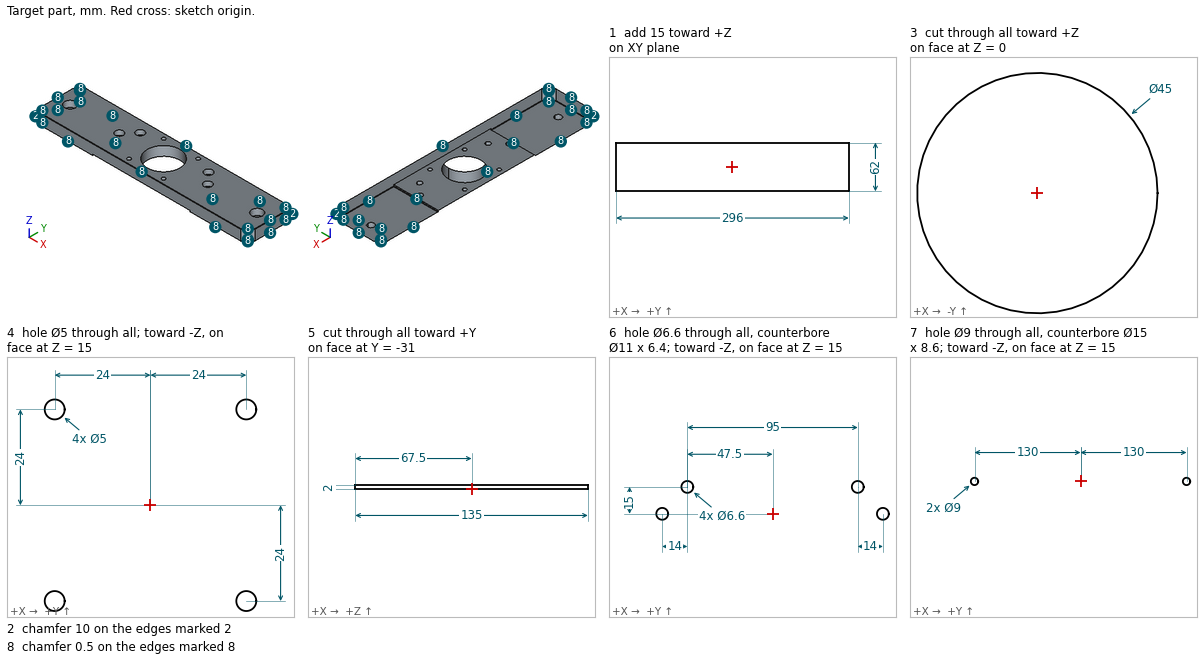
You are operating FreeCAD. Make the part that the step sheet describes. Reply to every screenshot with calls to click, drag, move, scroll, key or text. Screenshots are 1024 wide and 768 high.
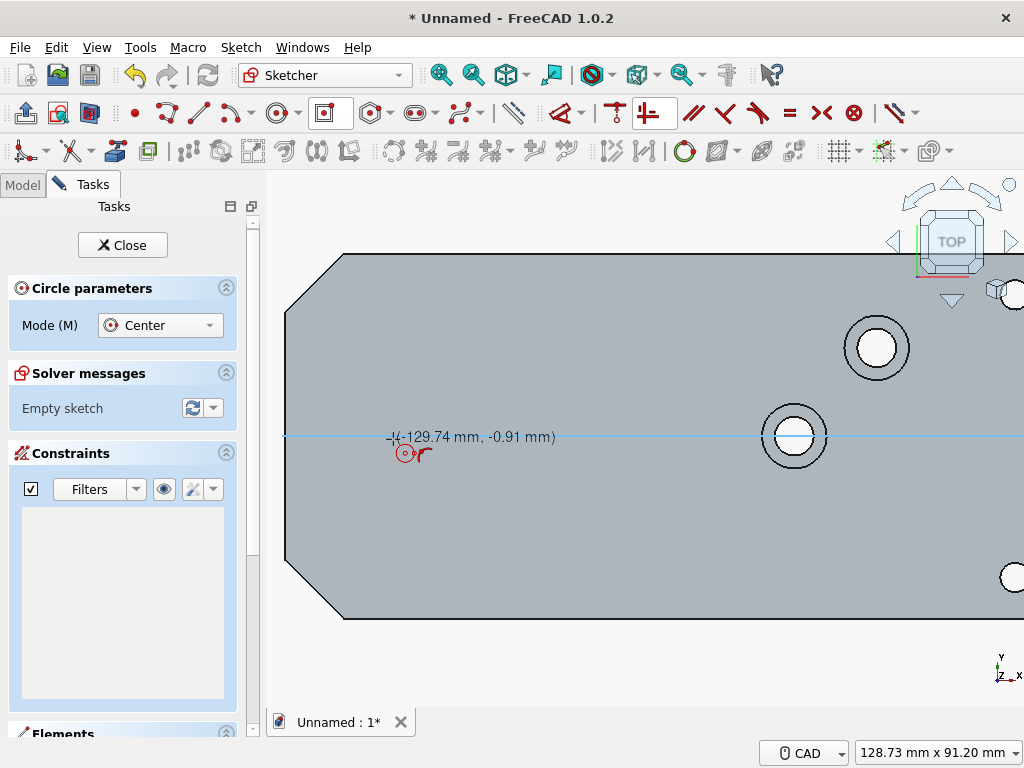
scroll(387, 439, down, 7)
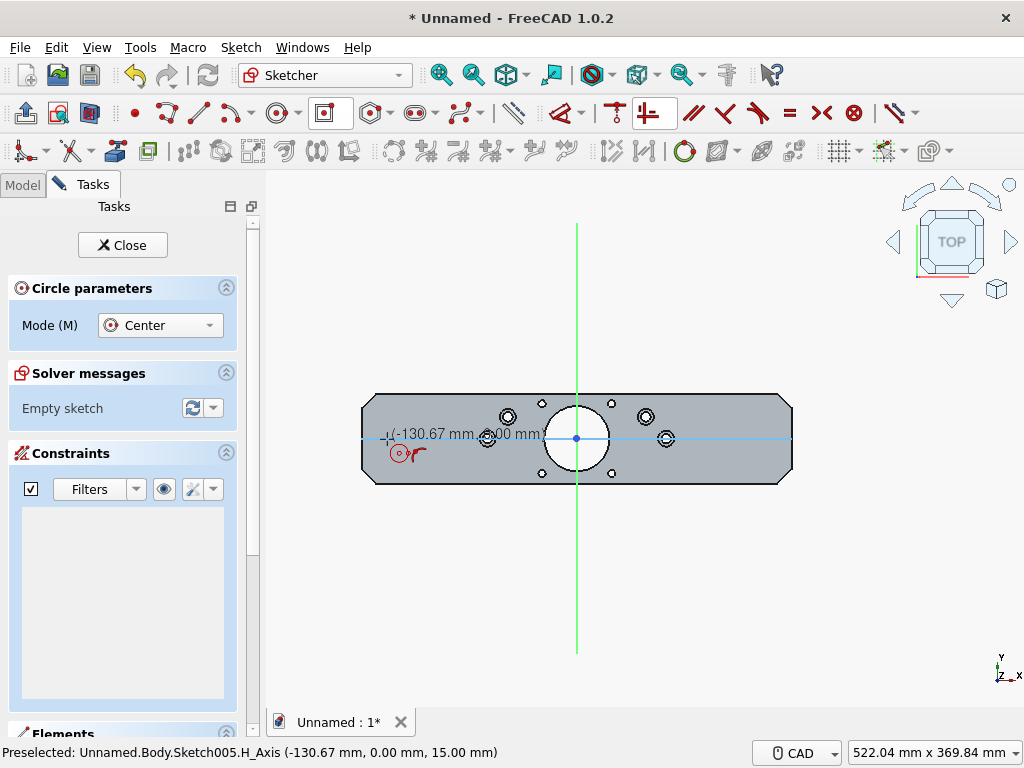
click(388, 439)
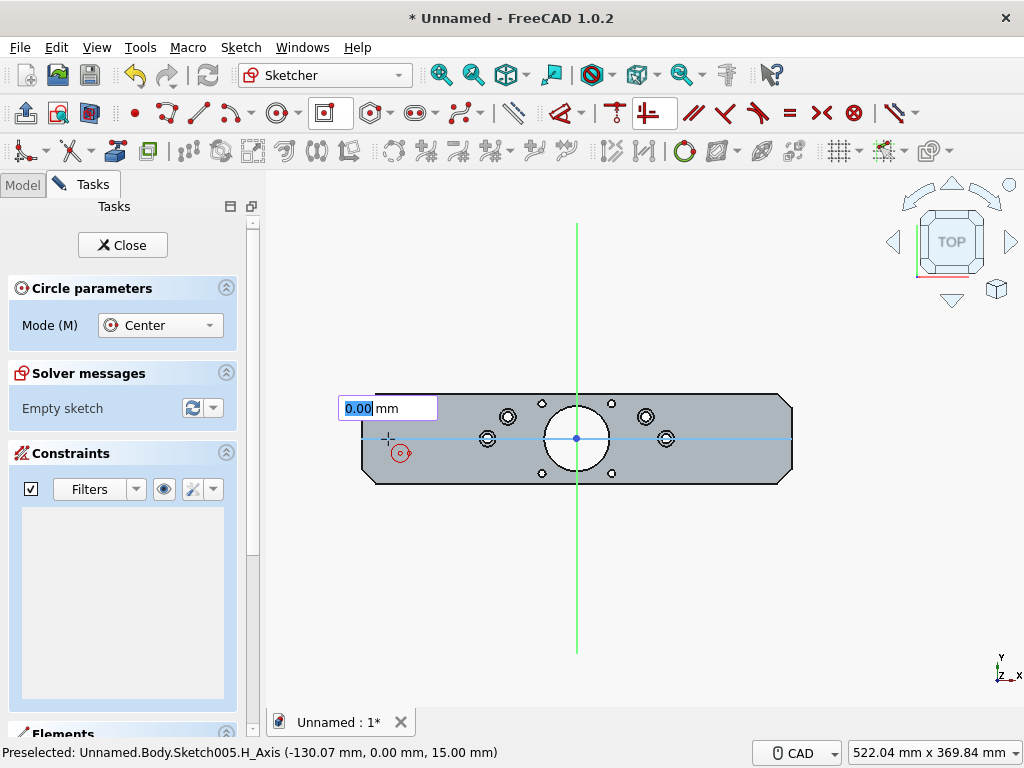
scroll(386, 445, up, 5)
move(385, 444)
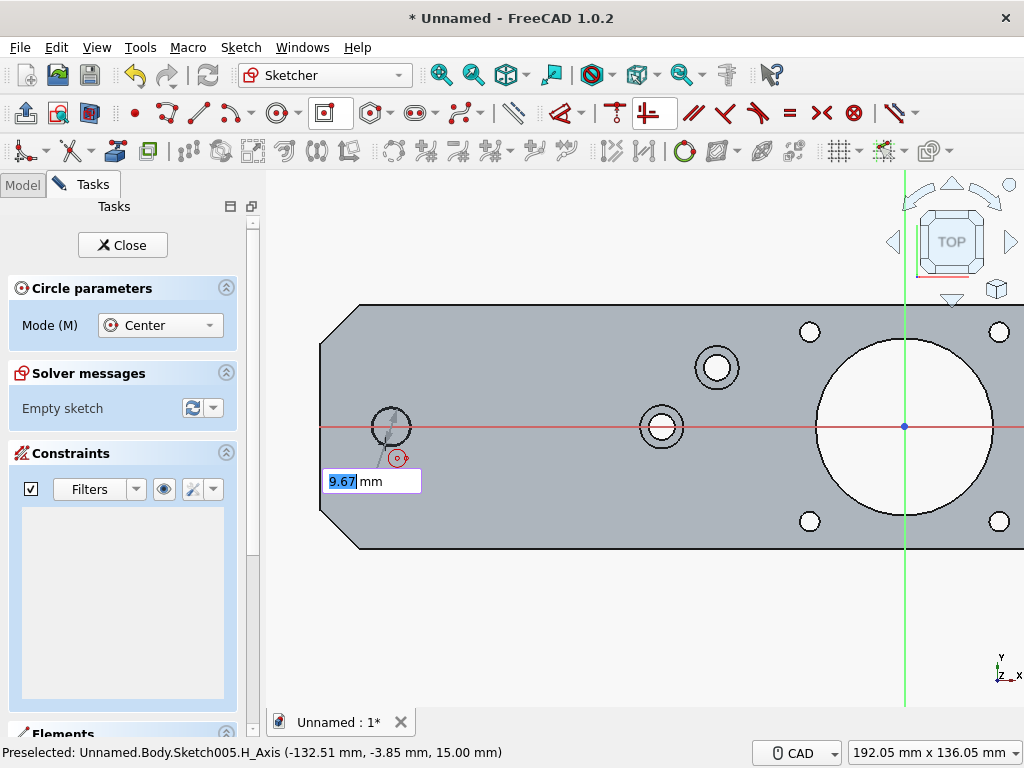
text(9)
key(Return)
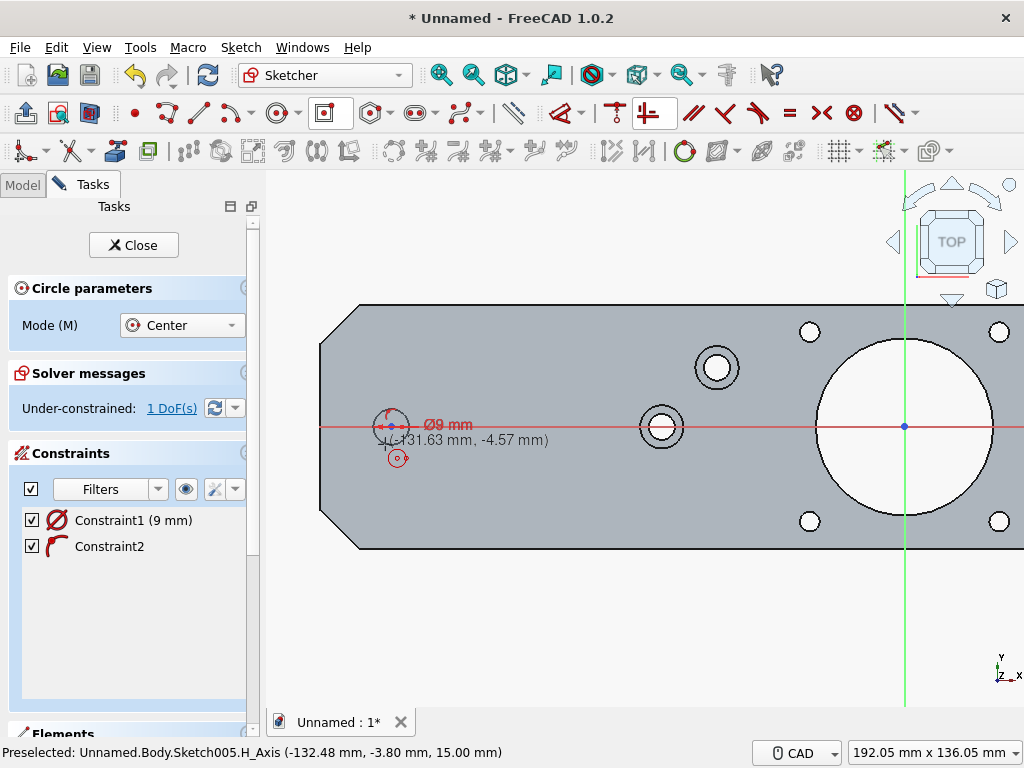
scroll(386, 445, down, 5)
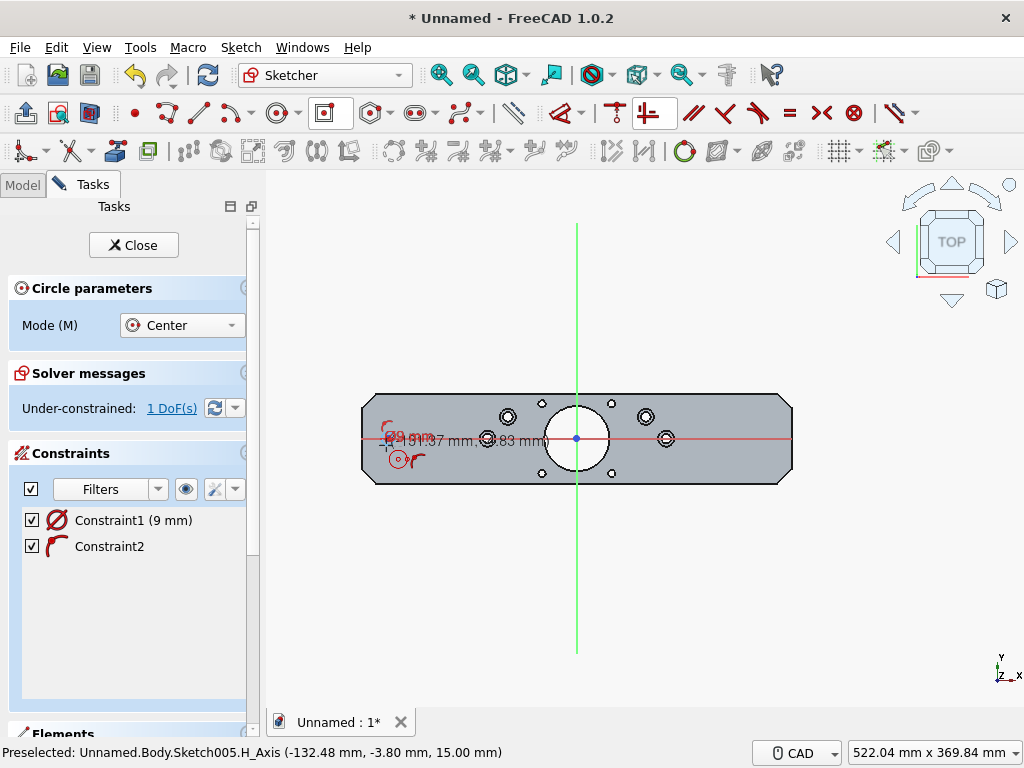
scroll(766, 439, up, 7)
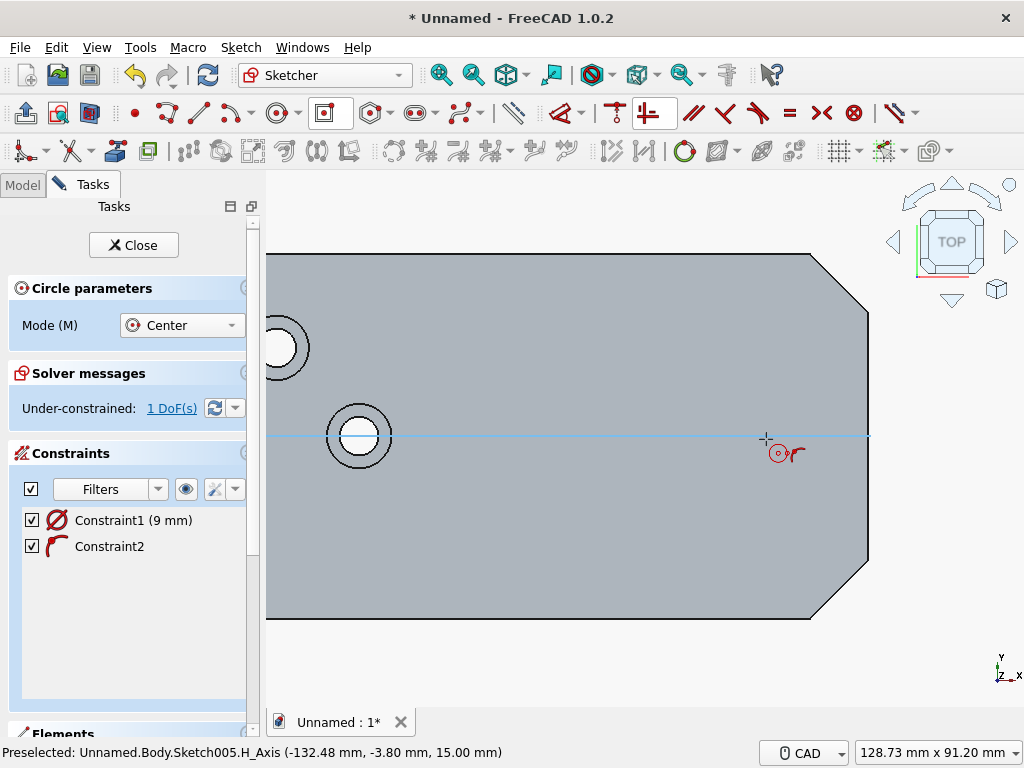
scroll(766, 439, down, 7)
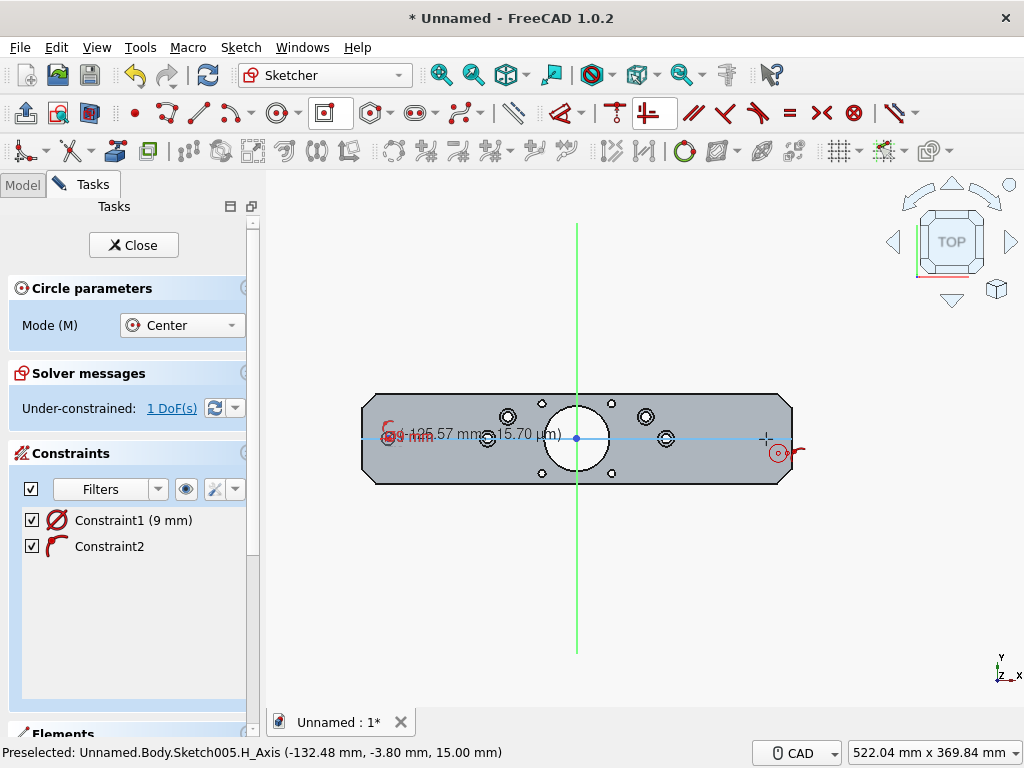
click(766, 439)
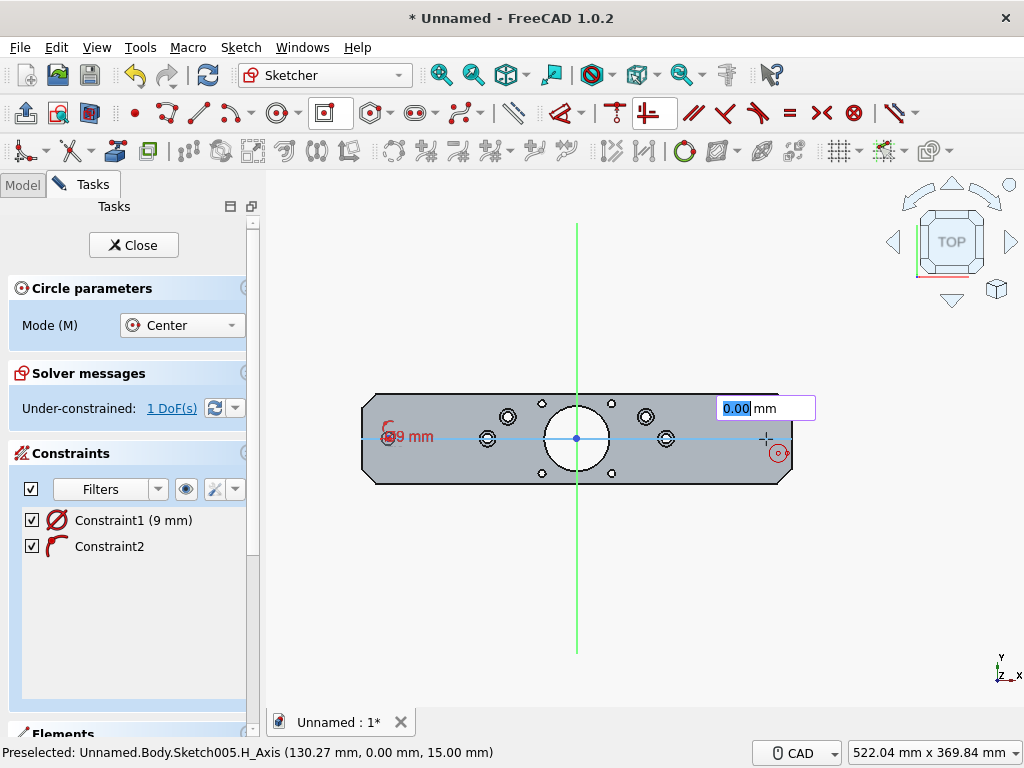
scroll(763, 445, up, 5)
move(763, 444)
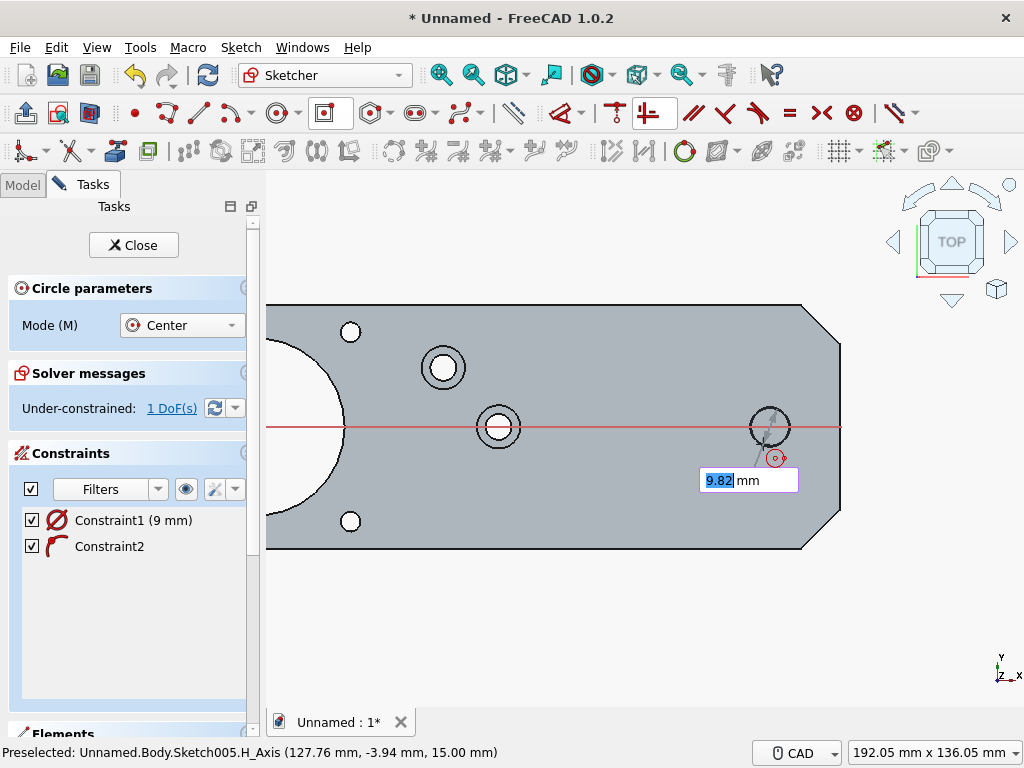
text(9)
key(Return)
key(Escape)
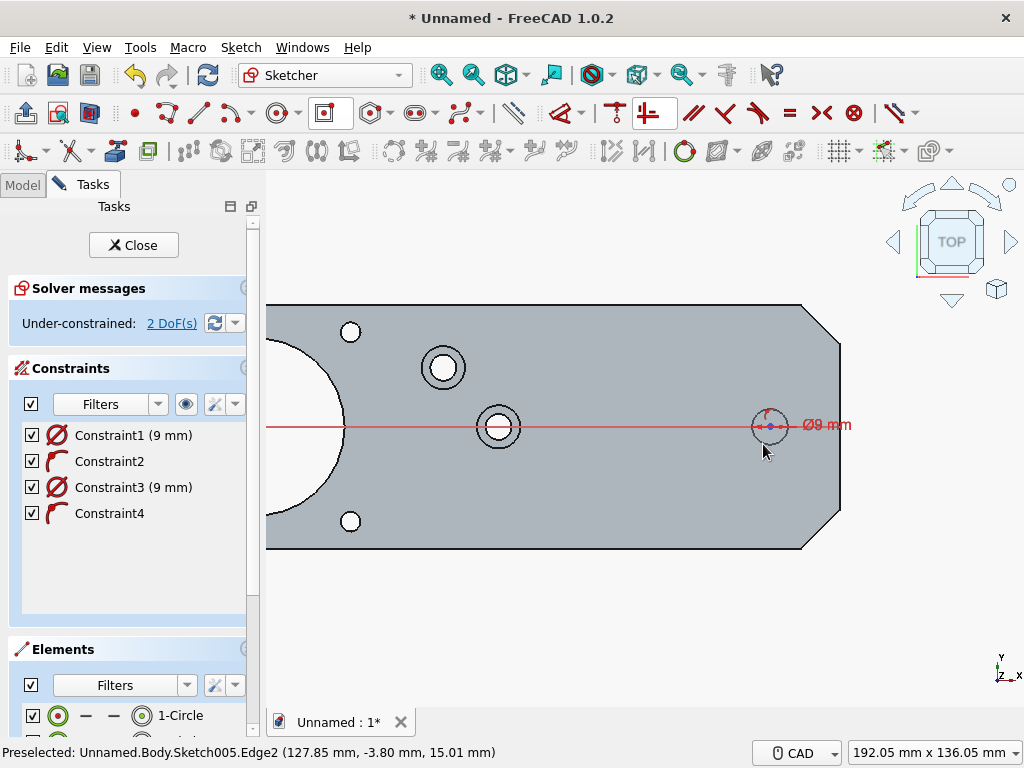
click(560, 114)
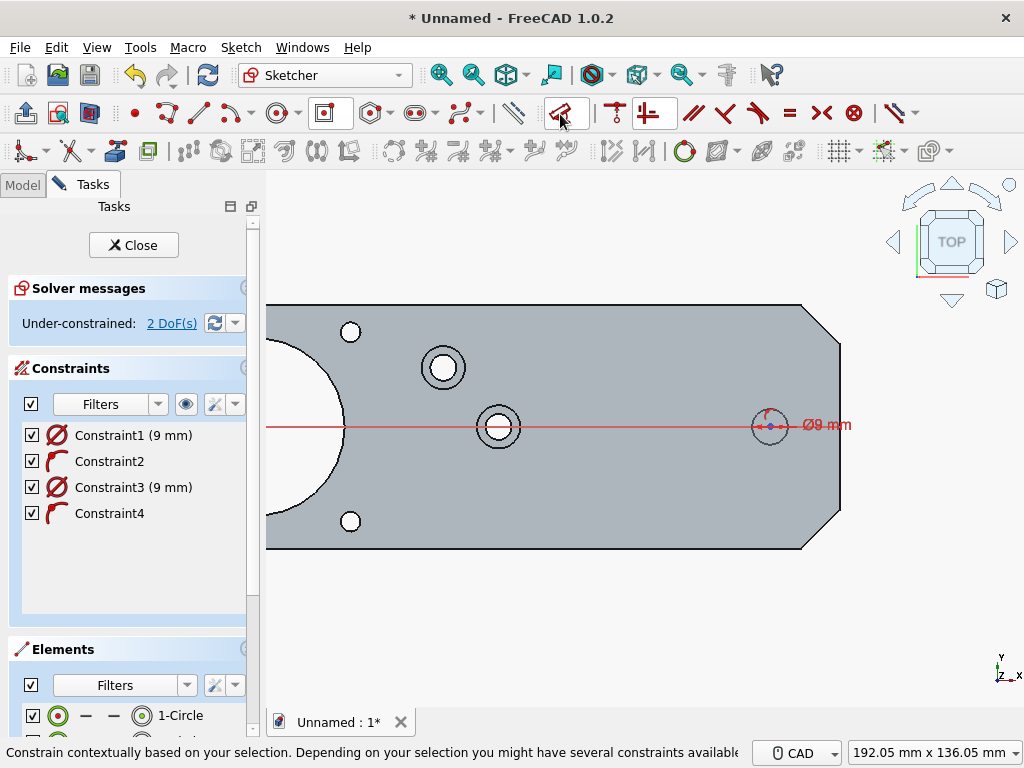
scroll(763, 445, down, 5)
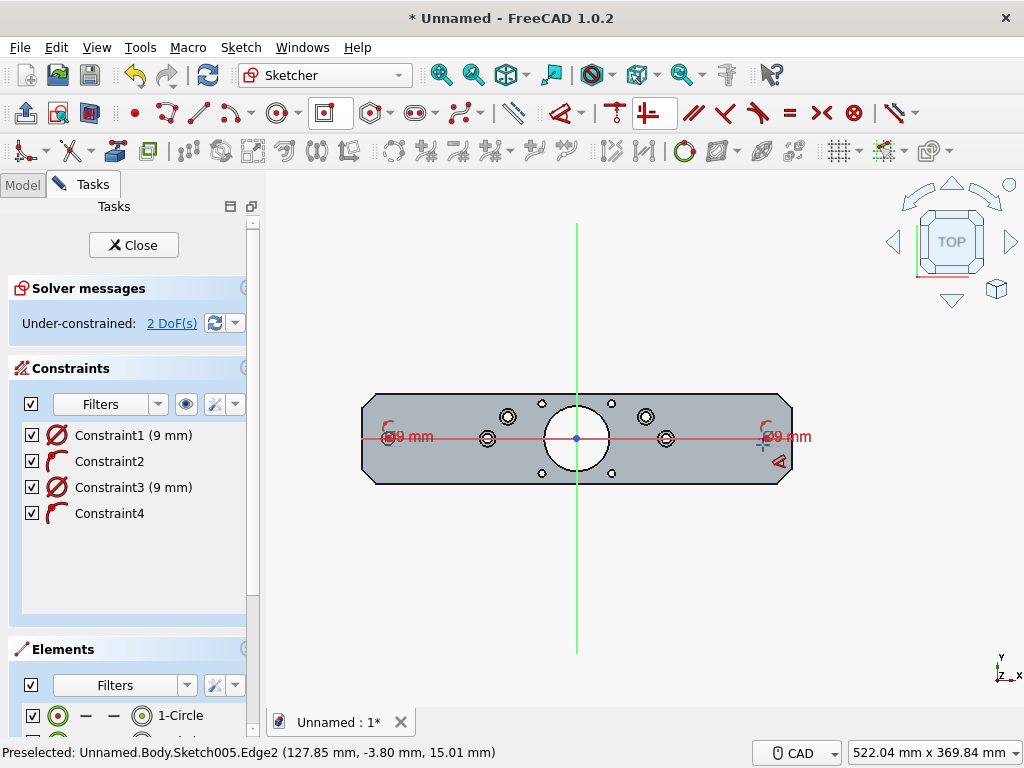
click(388, 439)
click(482, 473)